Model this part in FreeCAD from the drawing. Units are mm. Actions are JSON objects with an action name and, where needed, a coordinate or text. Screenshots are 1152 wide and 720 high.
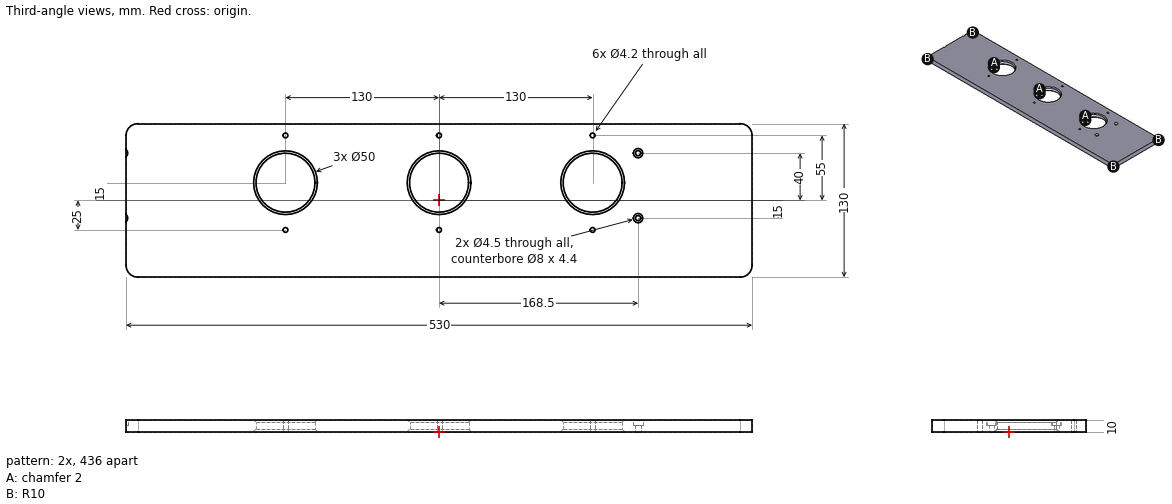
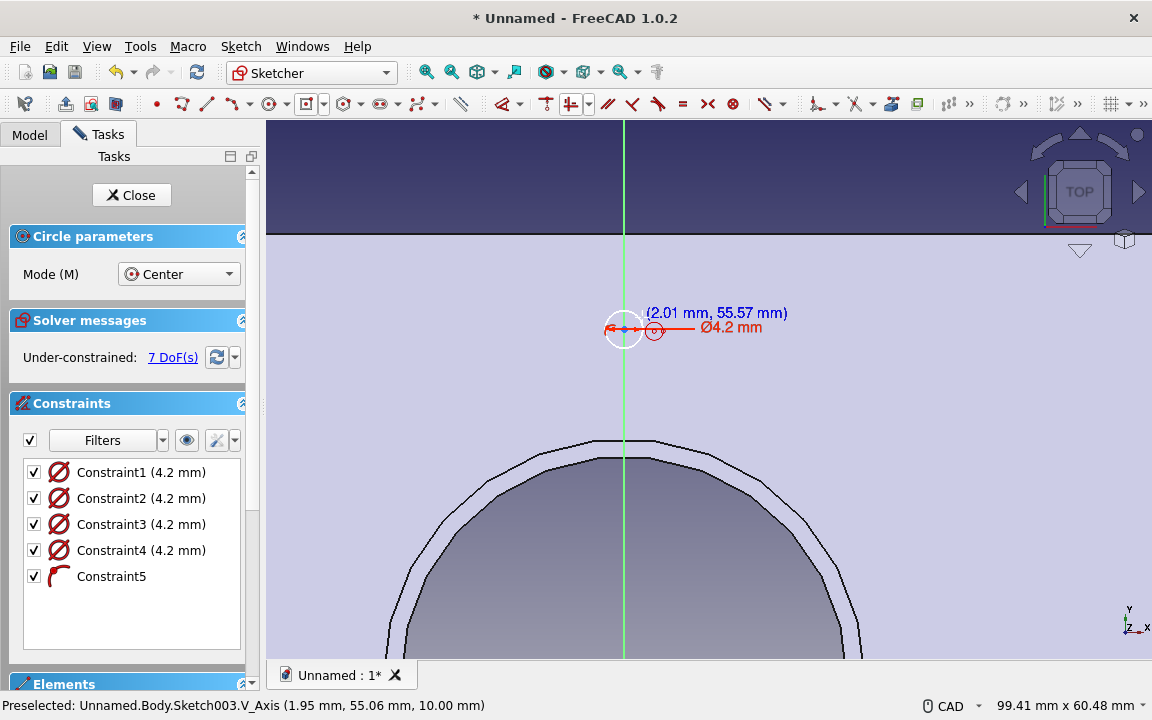
{"action": "scroll", "coordinate": [645, 316], "scroll_direction": "down", "scroll_amount": 8}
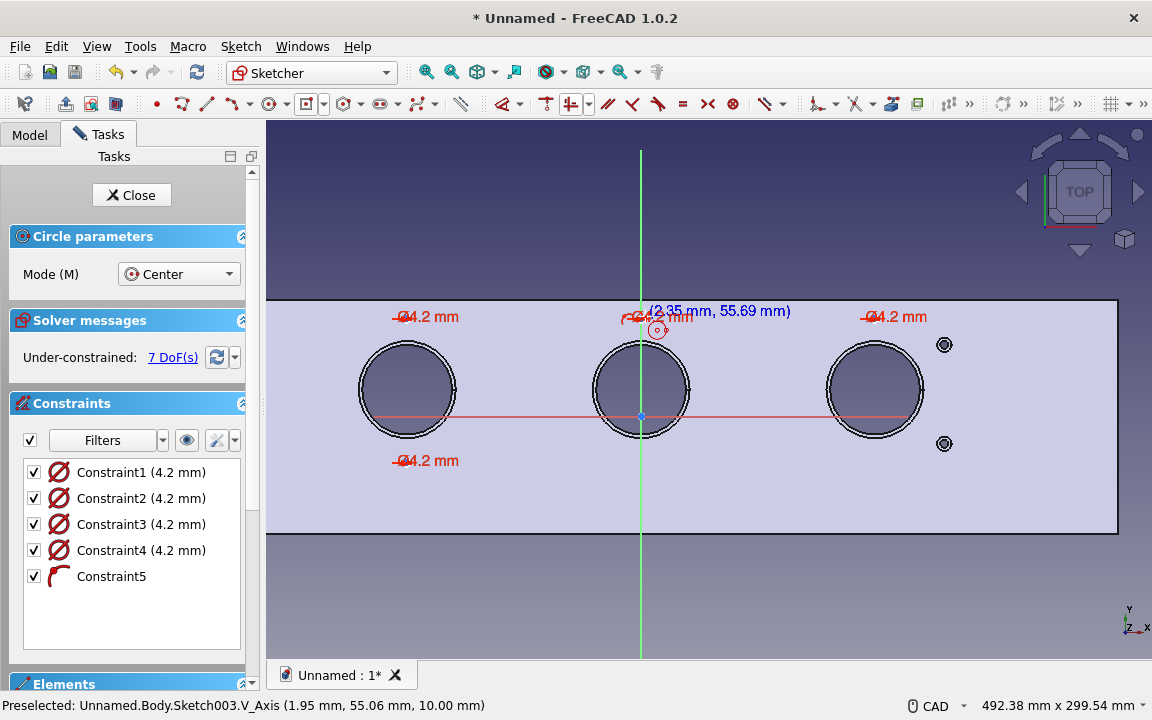
{"action": "scroll", "coordinate": [641, 462], "scroll_direction": "up", "scroll_amount": 9}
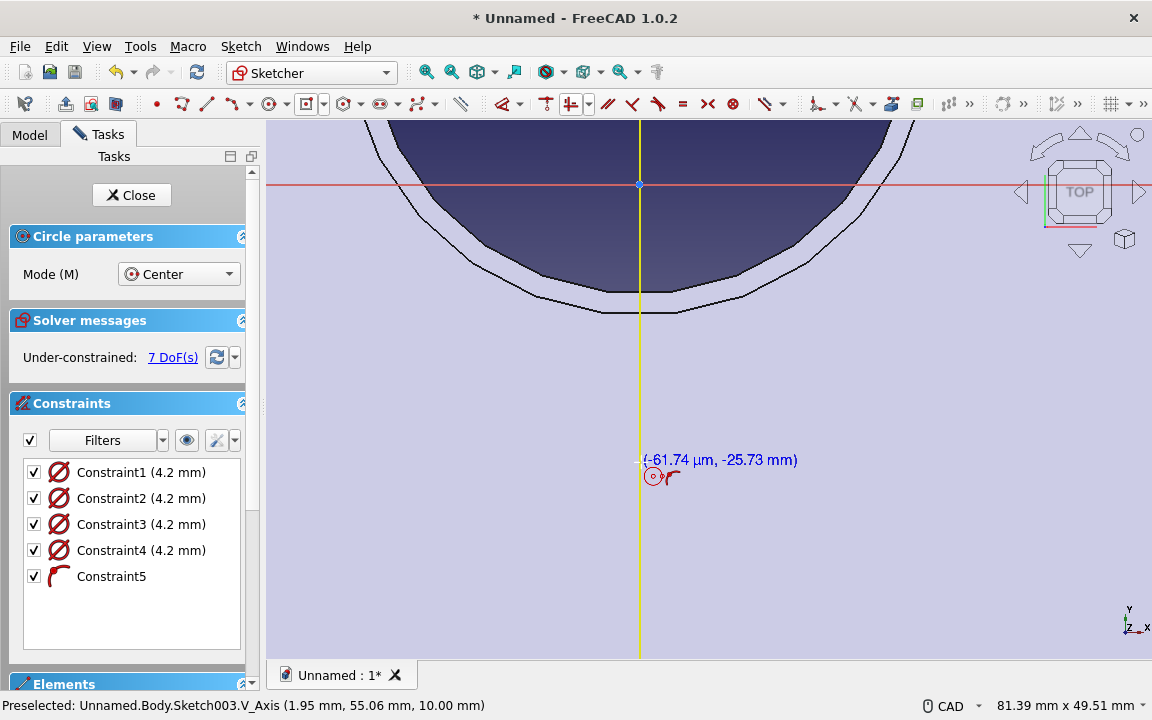
{"action": "scroll", "coordinate": [641, 462], "scroll_direction": "down", "scroll_amount": 9}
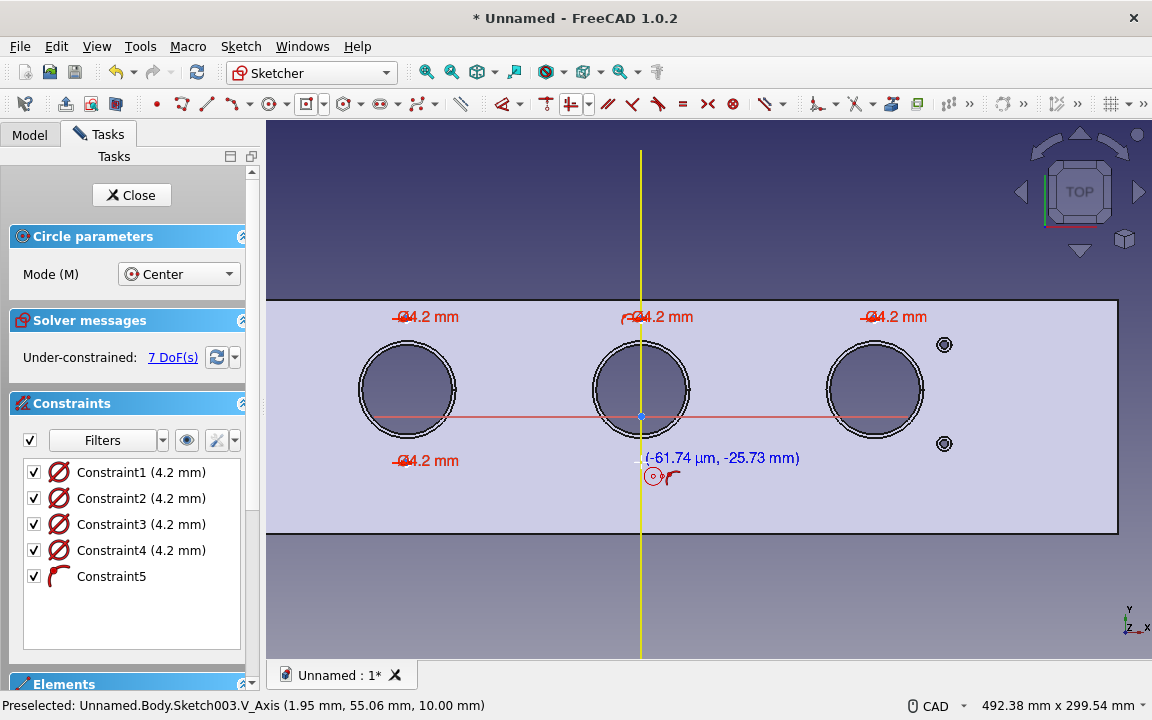
{"action": "left_click", "coordinate": [641, 462]}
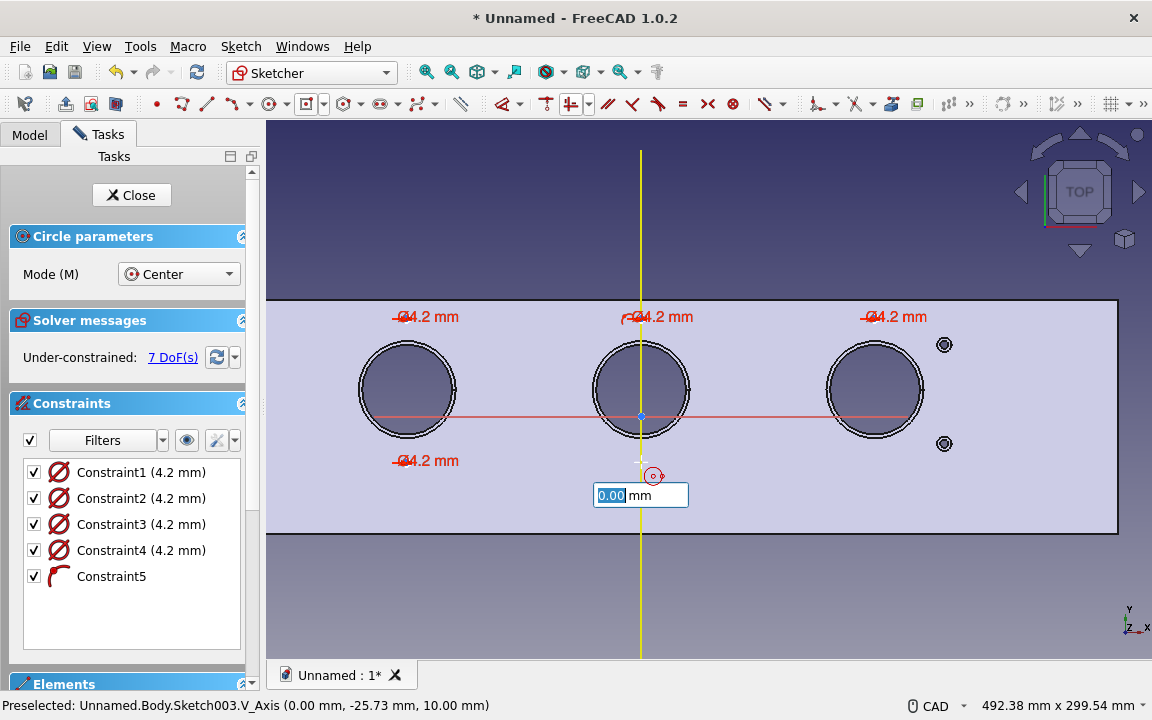
{"action": "scroll", "coordinate": [645, 460], "scroll_direction": "up", "scroll_amount": 8}
{"action": "mouse_move", "coordinate": [642, 459]}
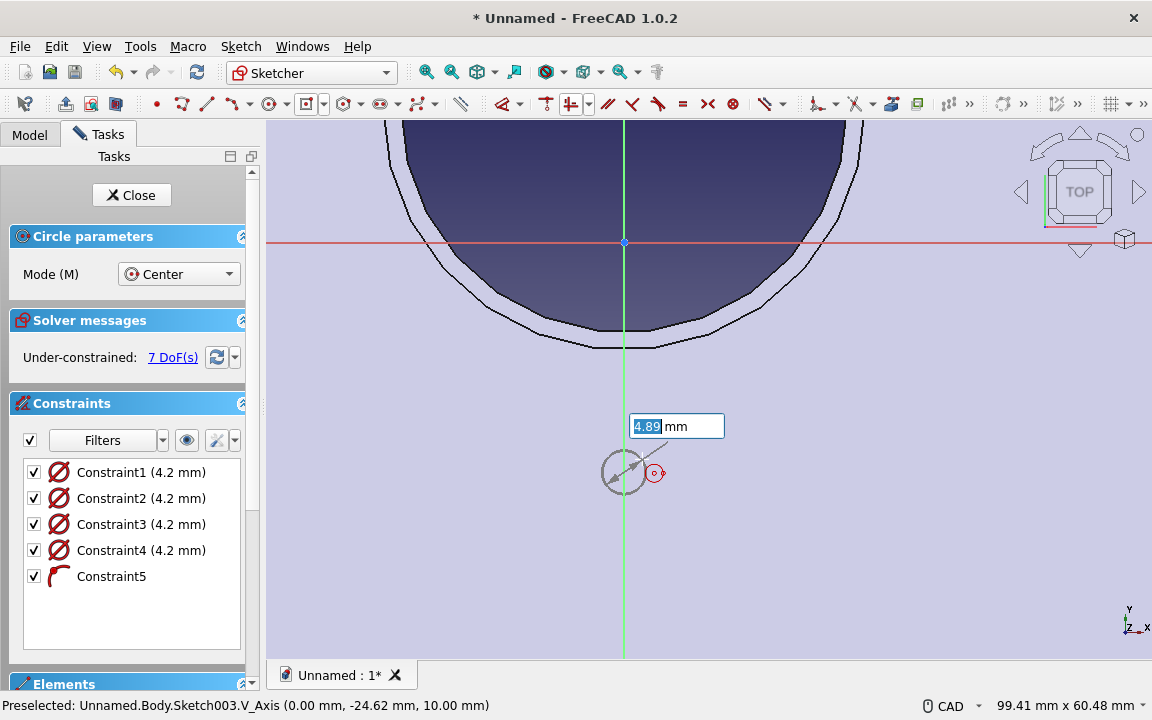
{"action": "type", "text": "4.2"}
{"action": "key", "text": "Return"}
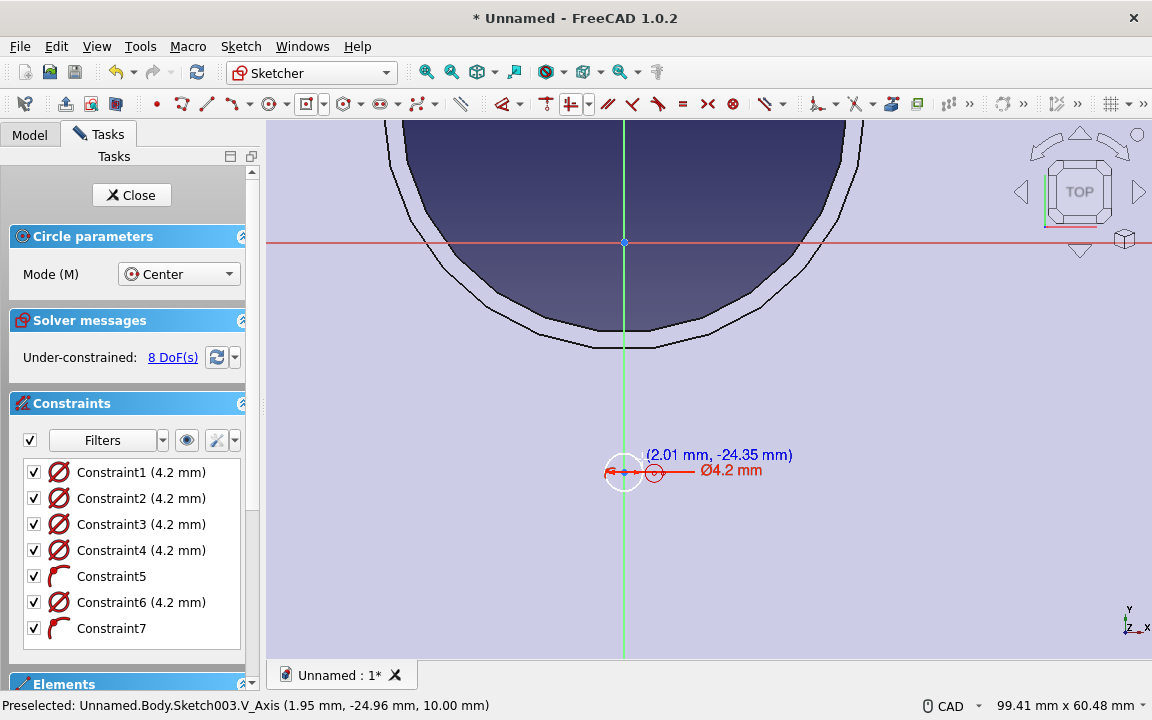
{"action": "scroll", "coordinate": [645, 460], "scroll_direction": "down", "scroll_amount": 8}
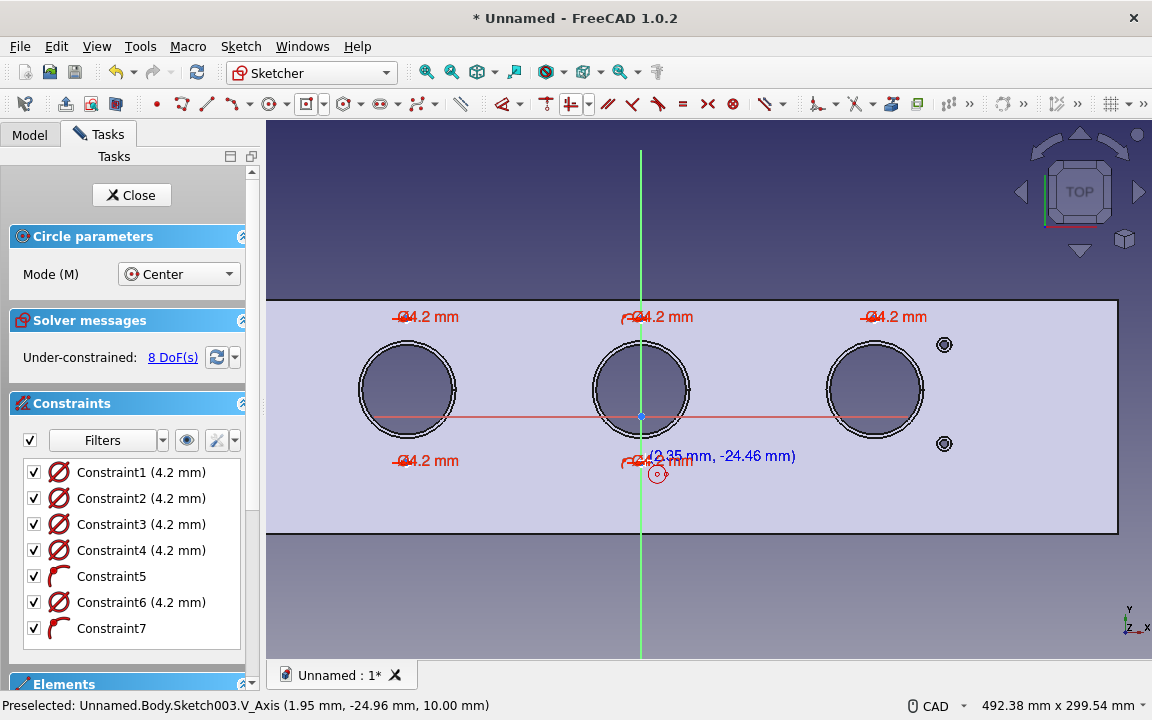
{"action": "scroll", "coordinate": [875, 462], "scroll_direction": "up", "scroll_amount": 9}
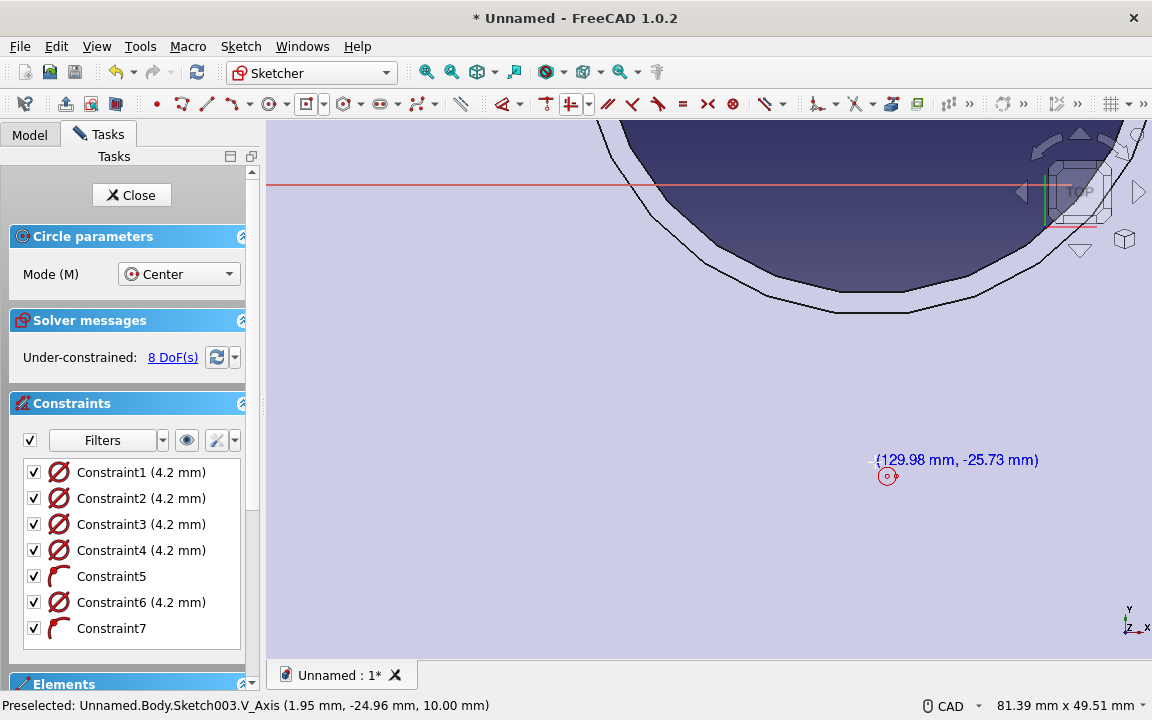
{"action": "scroll", "coordinate": [875, 462], "scroll_direction": "down", "scroll_amount": 9}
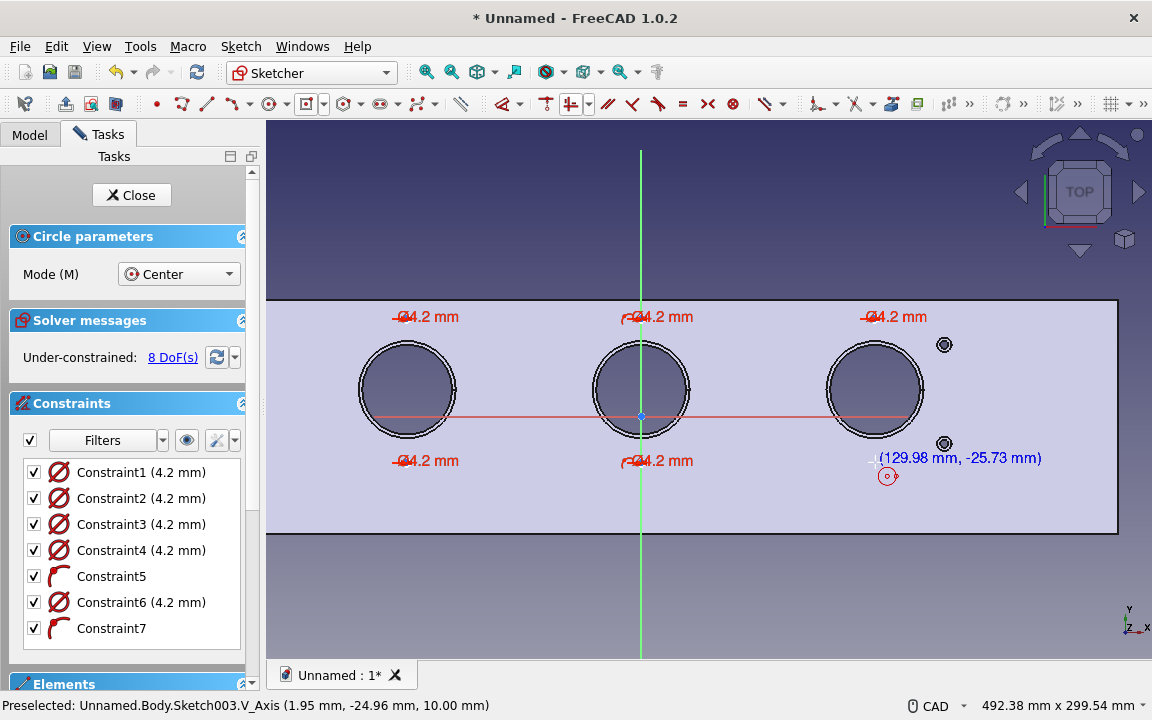
{"action": "left_click", "coordinate": [875, 462]}
{"action": "mouse_move", "coordinate": [878, 459]}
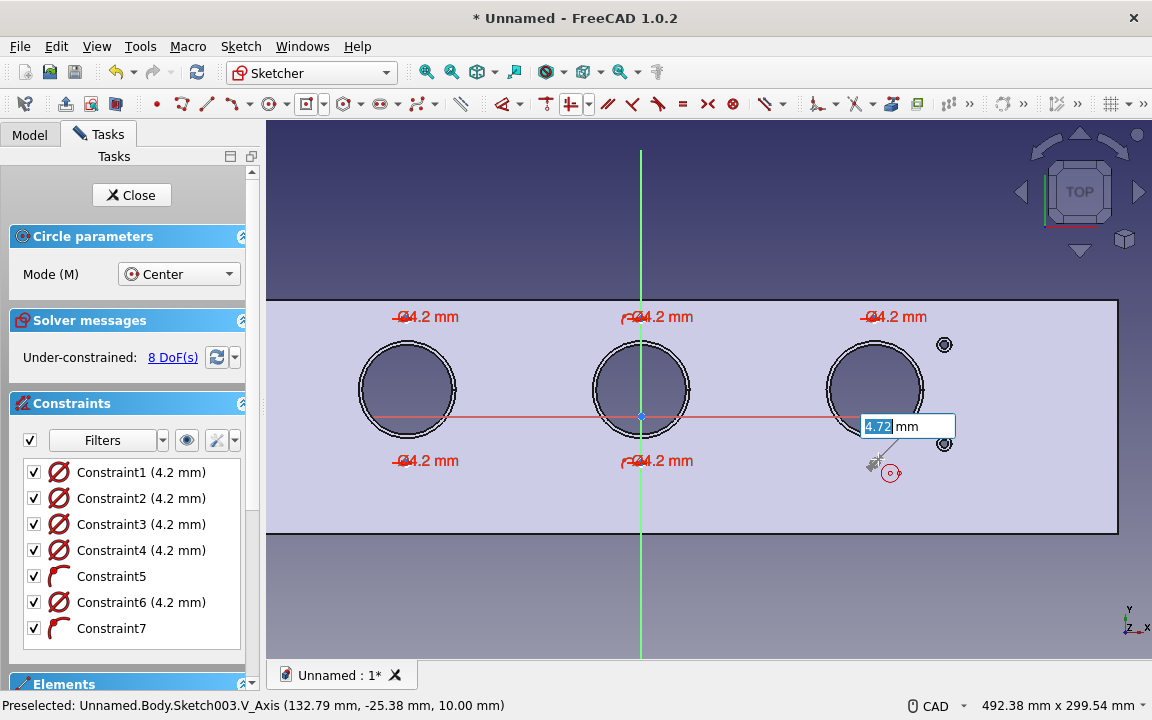
{"action": "type", "text": "4.2"}
{"action": "key", "text": "Return"}
{"action": "key", "text": "Escape"}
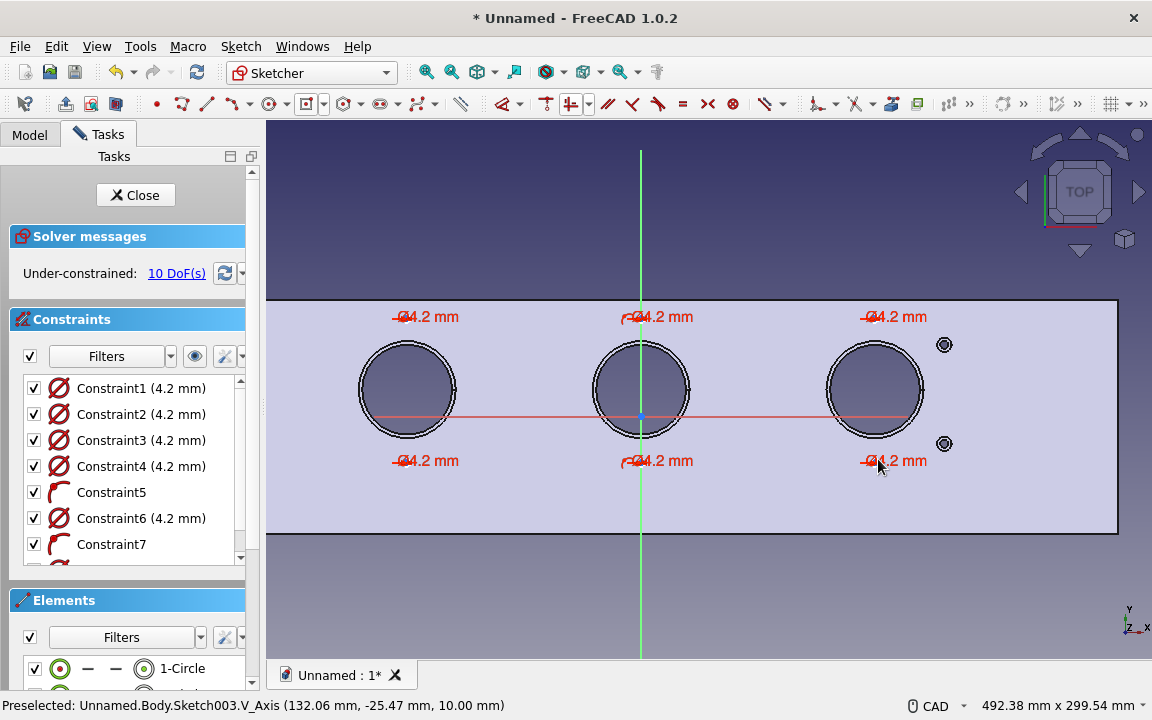
{"action": "left_click", "coordinate": [407, 463]}